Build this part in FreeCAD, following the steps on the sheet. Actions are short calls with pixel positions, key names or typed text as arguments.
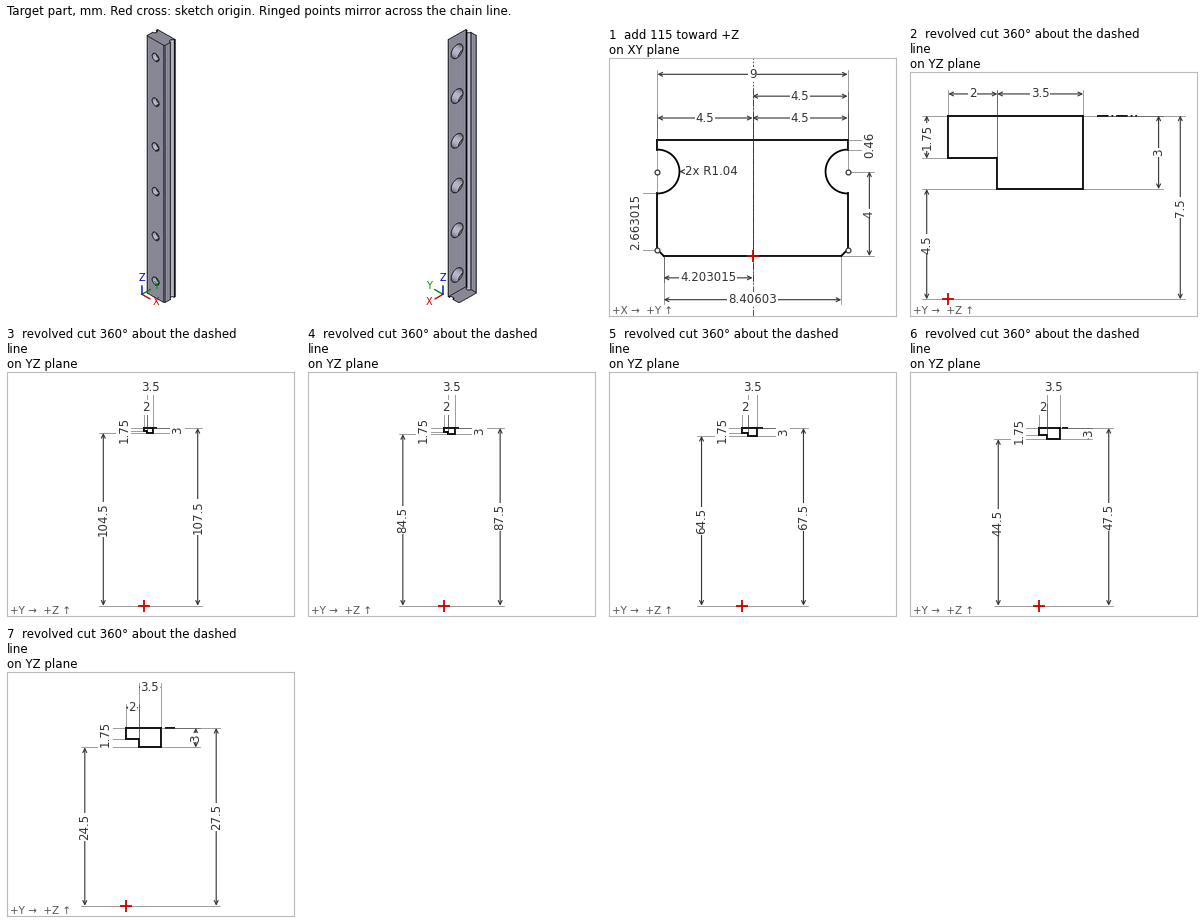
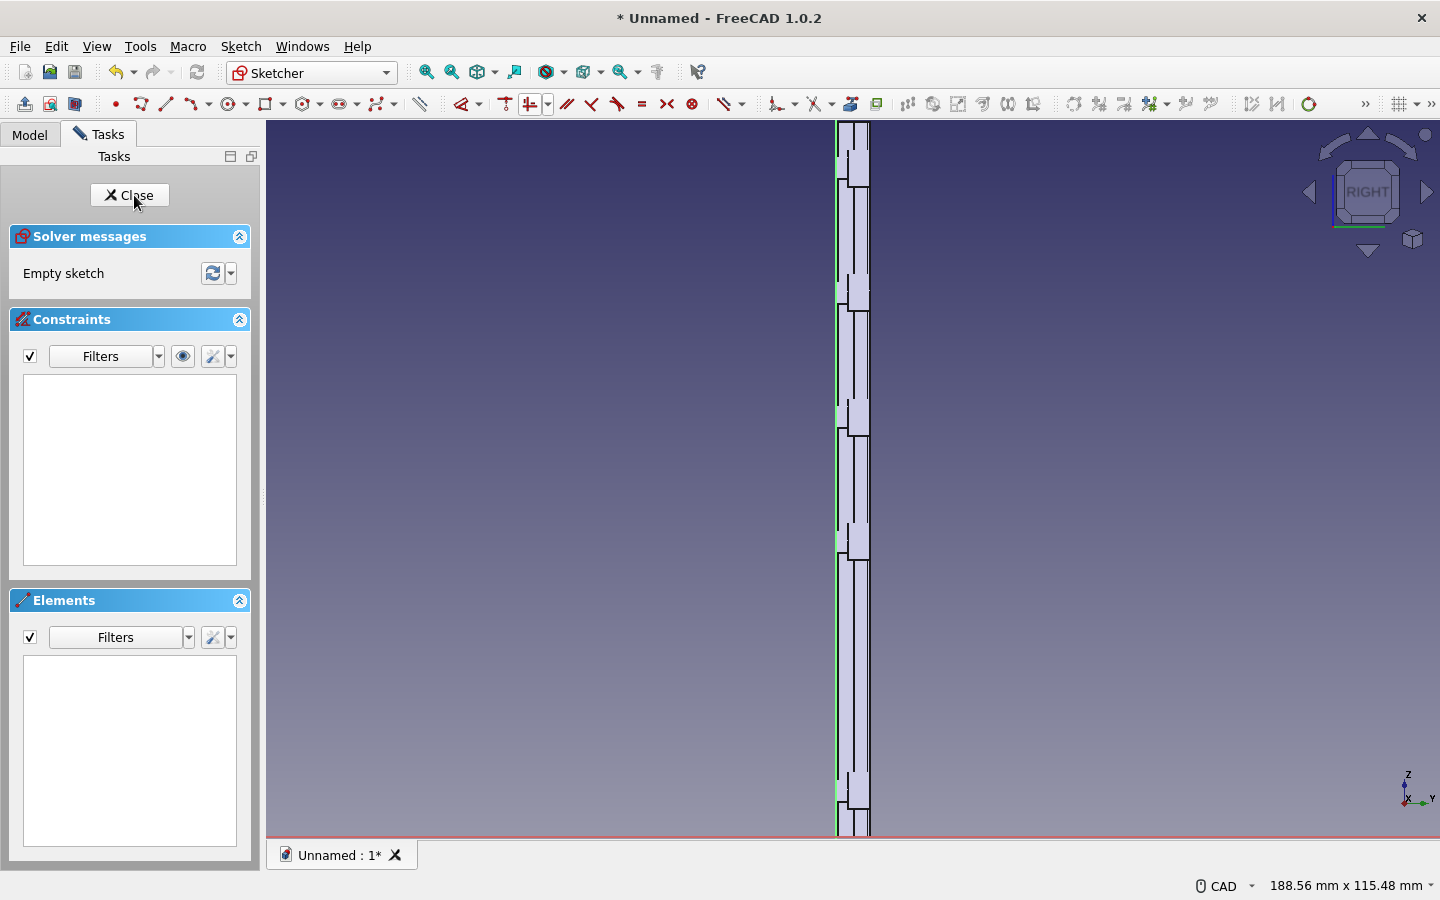
scroll(866, 691, up, 13)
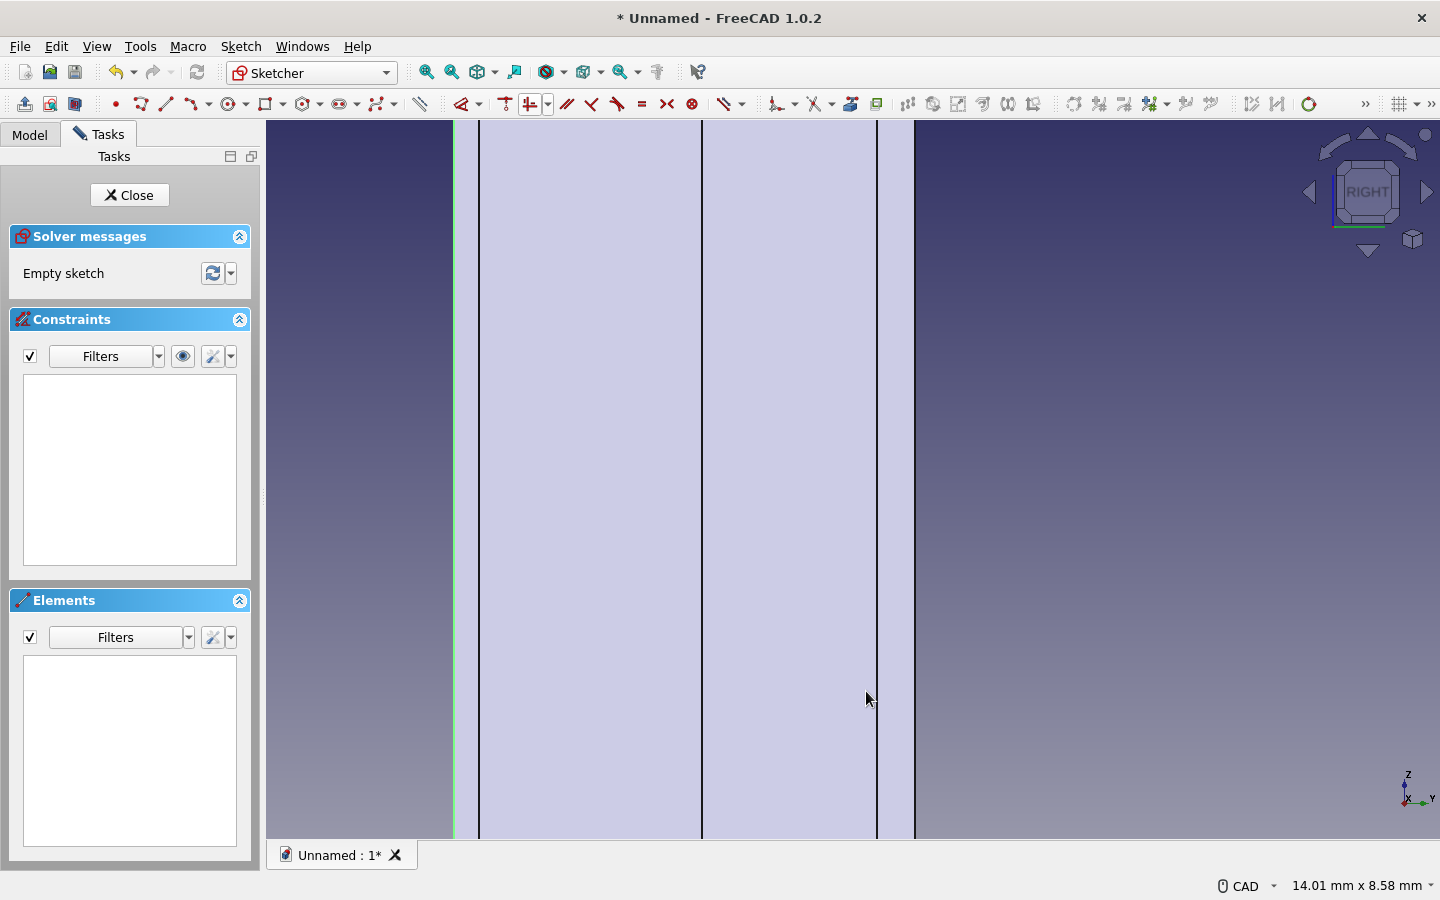
click(141, 104)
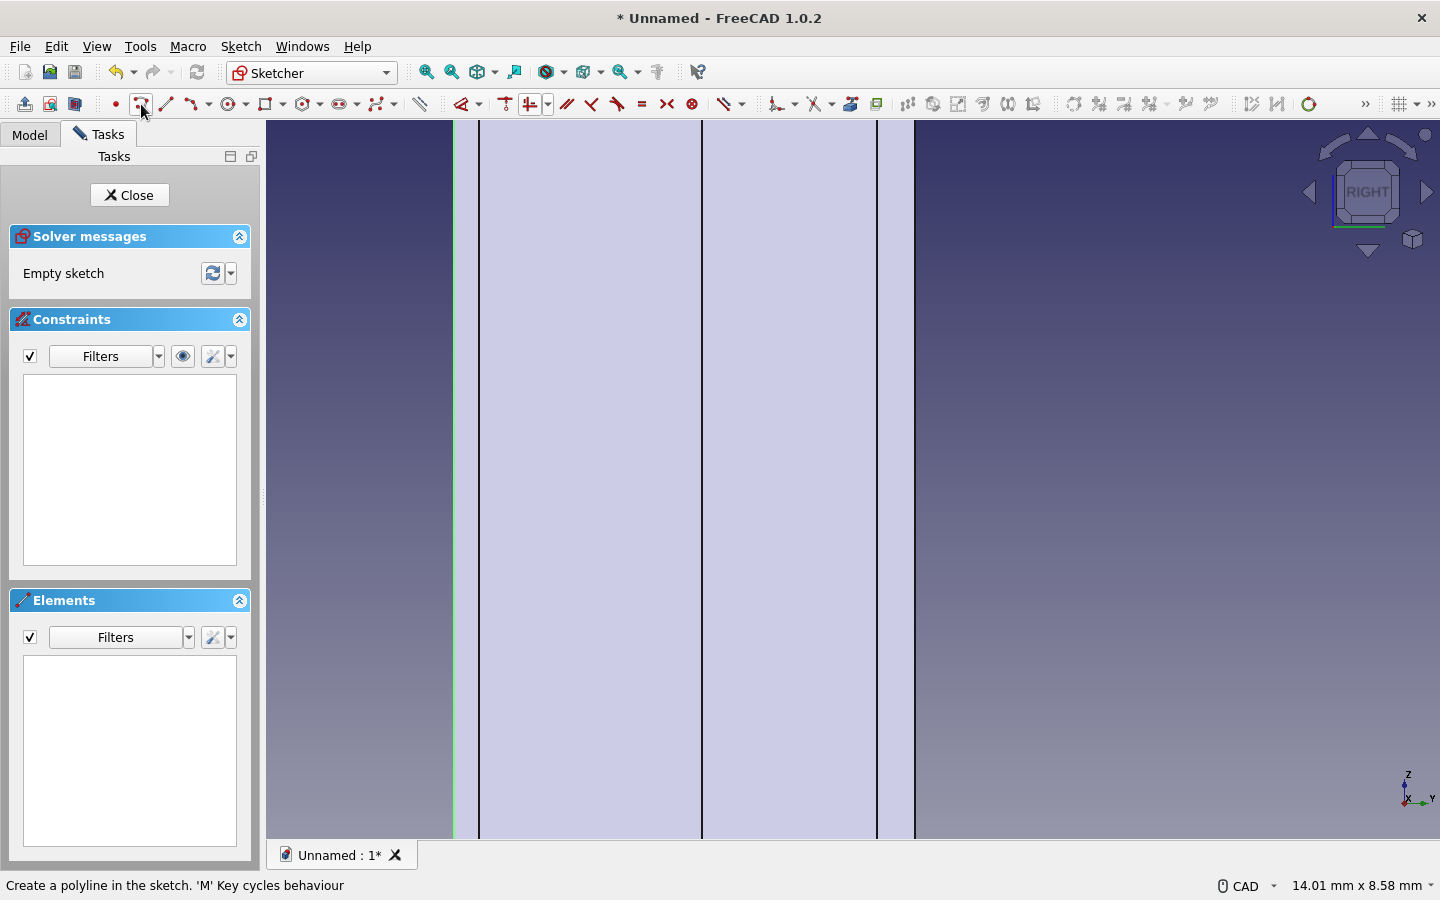
click(622, 600)
click(915, 600)
click(915, 348)
click(454, 348)
click(463, 495)
click(622, 495)
click(622, 601)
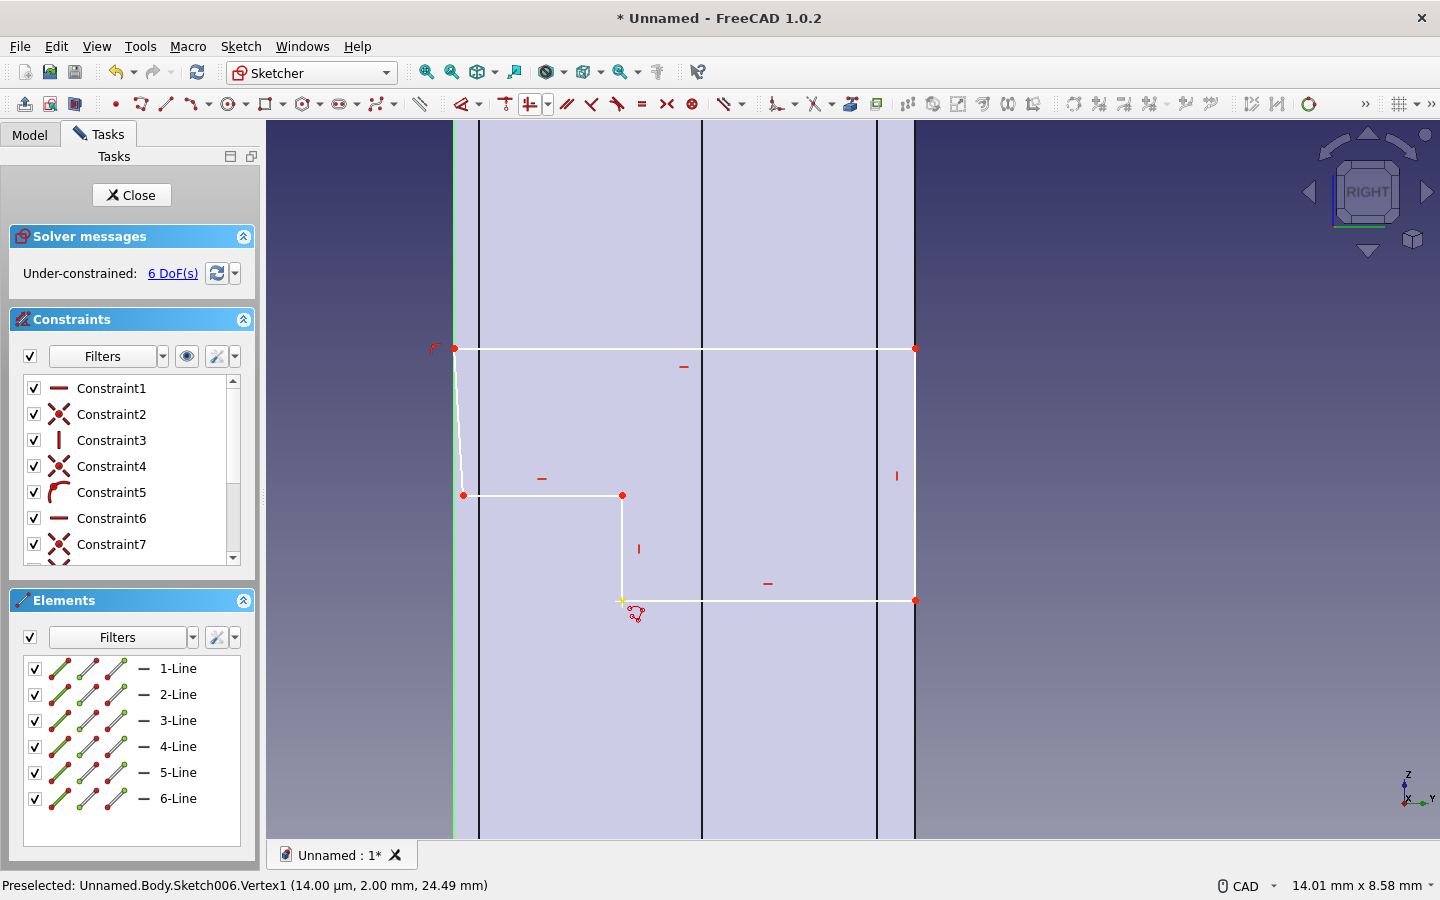
key(g)
key(l)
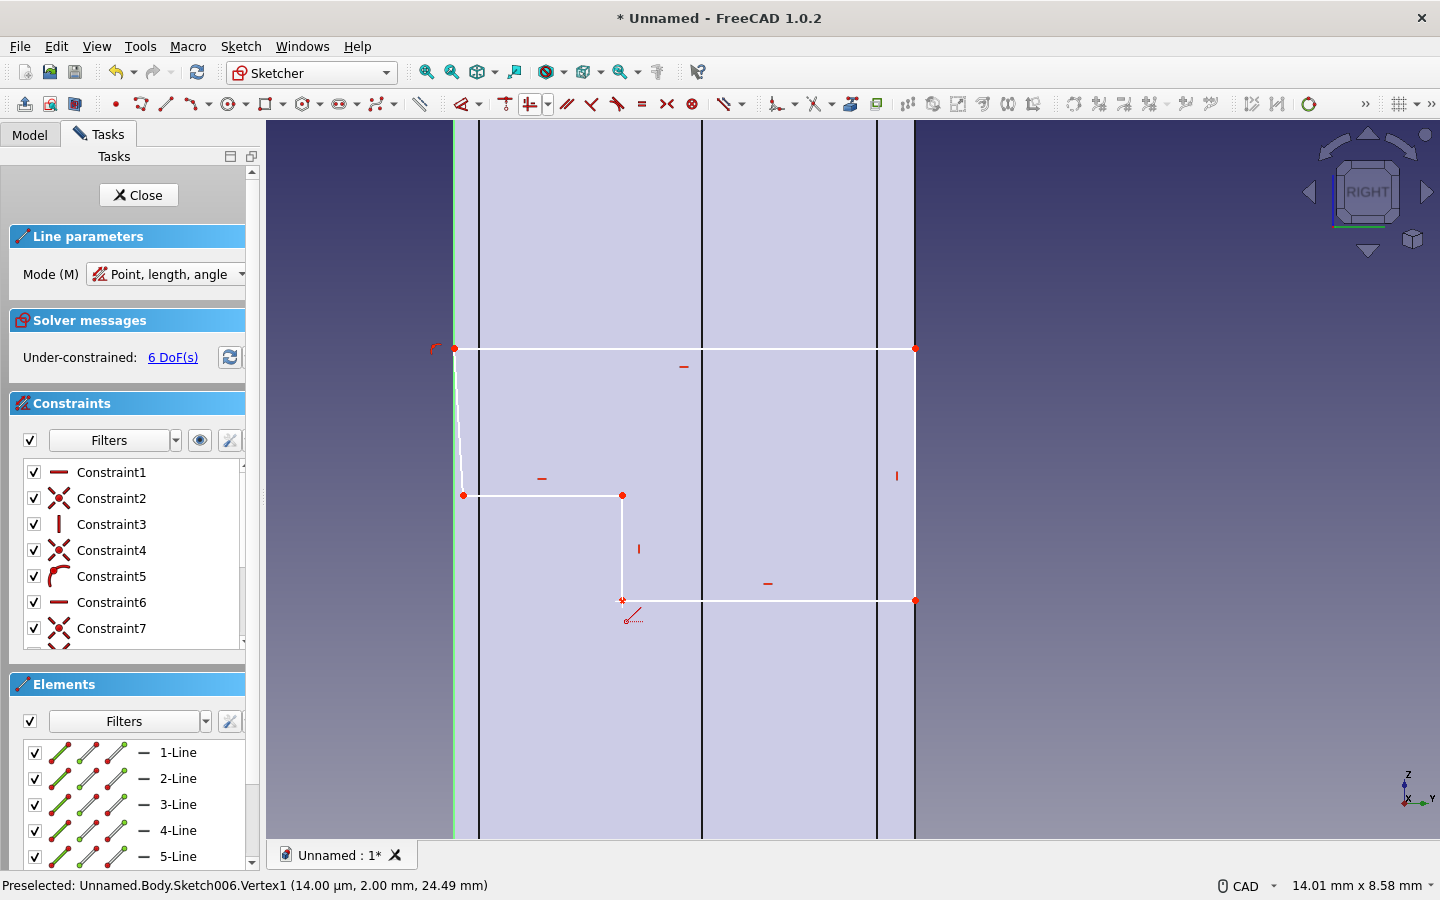
click(961, 348)
click(1100, 348)
key(Escape)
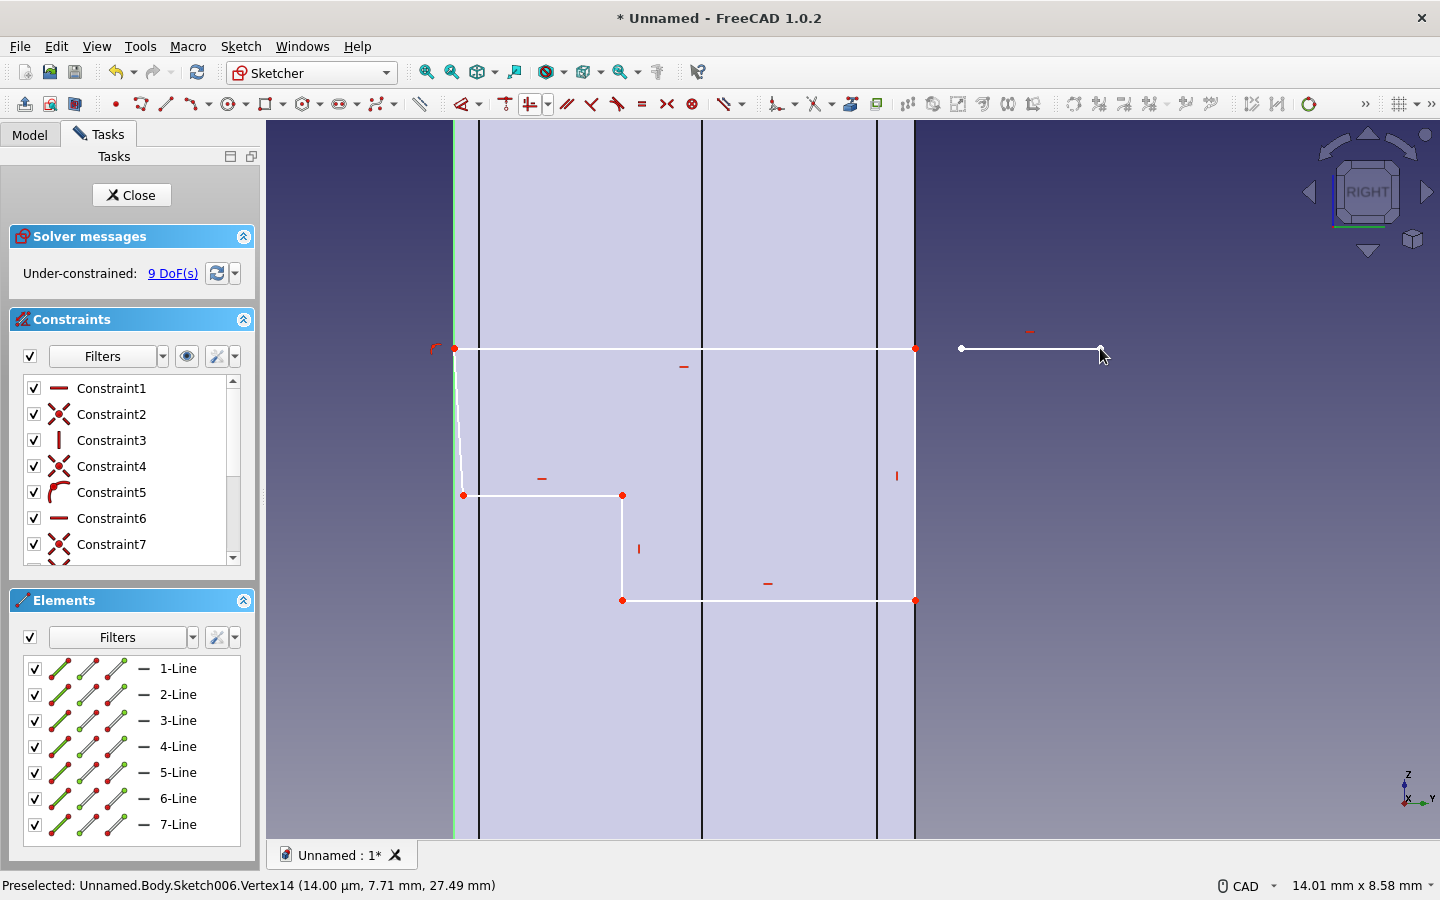
click(1003, 349)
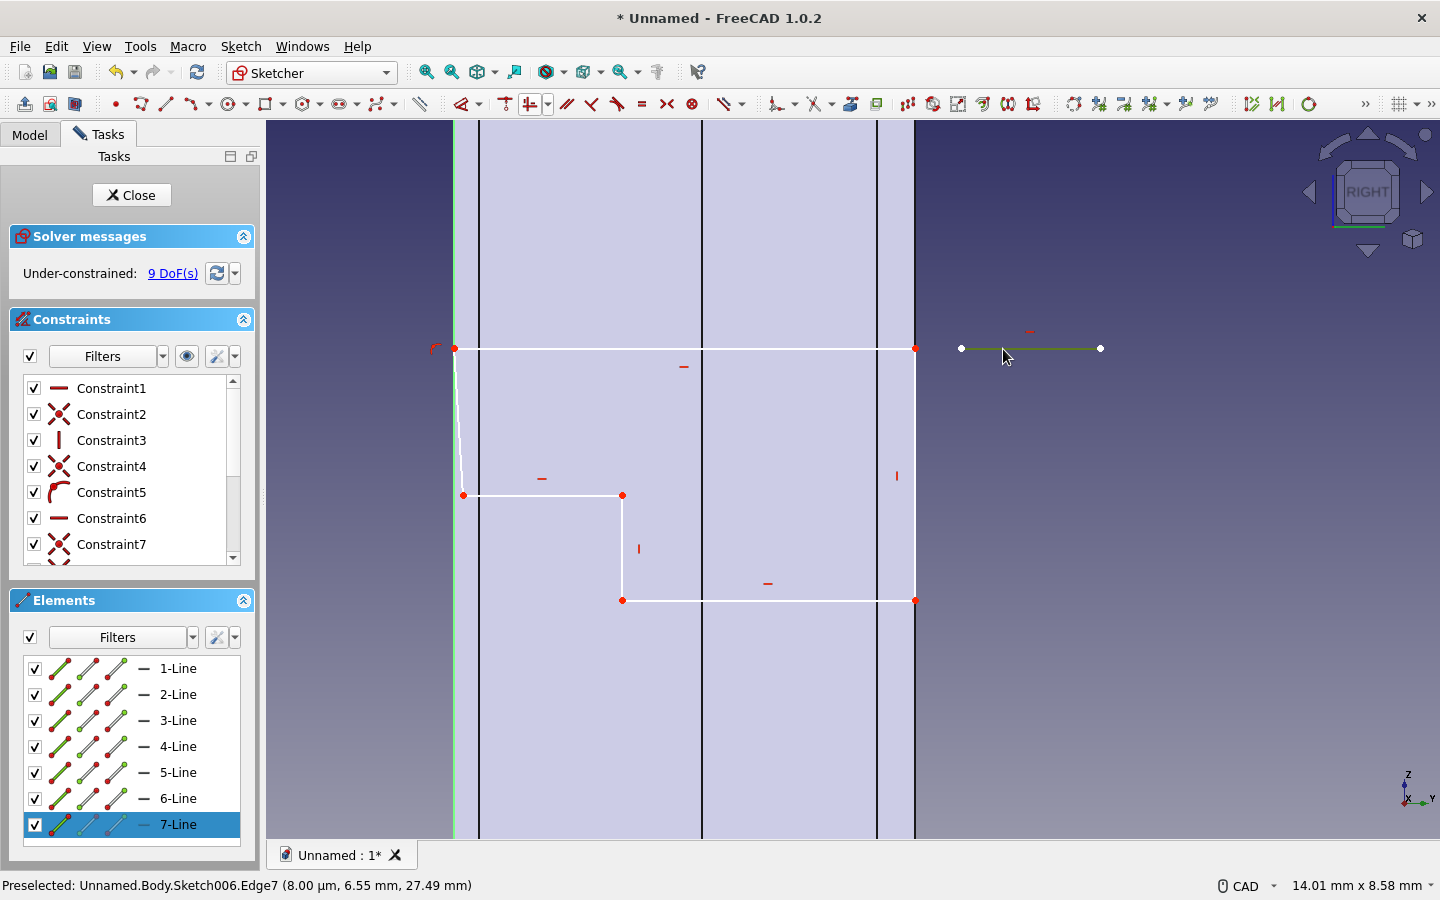
key(g)
key(n)